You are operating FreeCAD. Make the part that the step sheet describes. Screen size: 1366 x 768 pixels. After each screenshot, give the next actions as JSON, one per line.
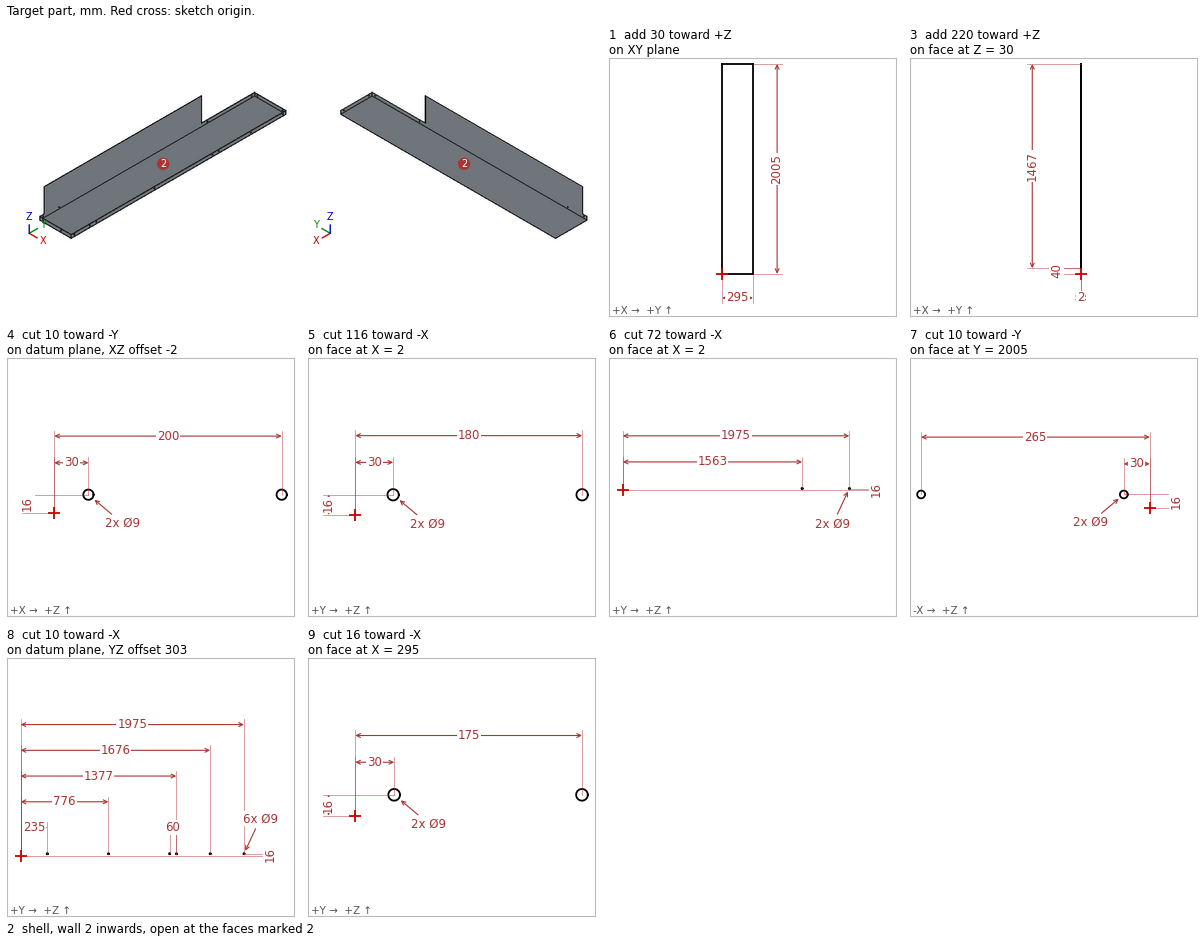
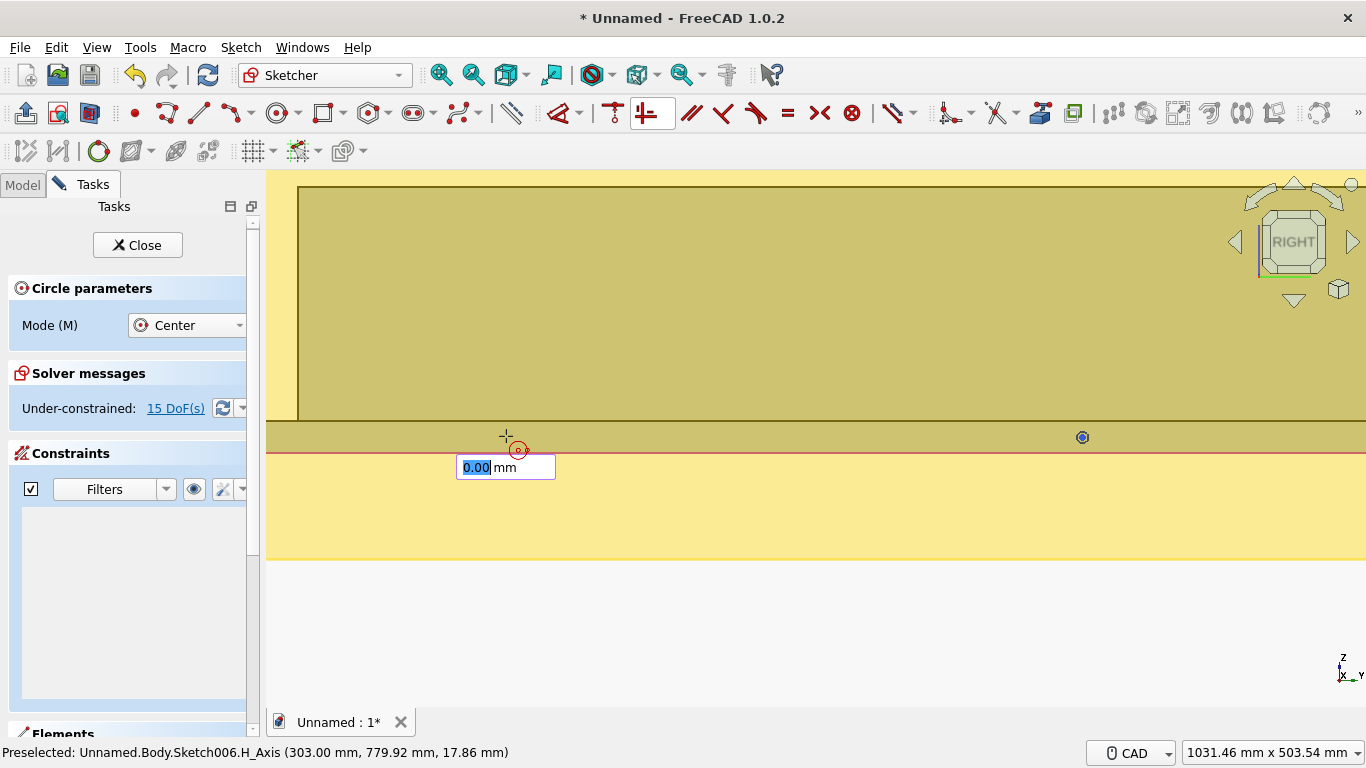
{"action": "scroll", "coordinate": [510, 433], "scroll_direction": "up", "scroll_amount": 6}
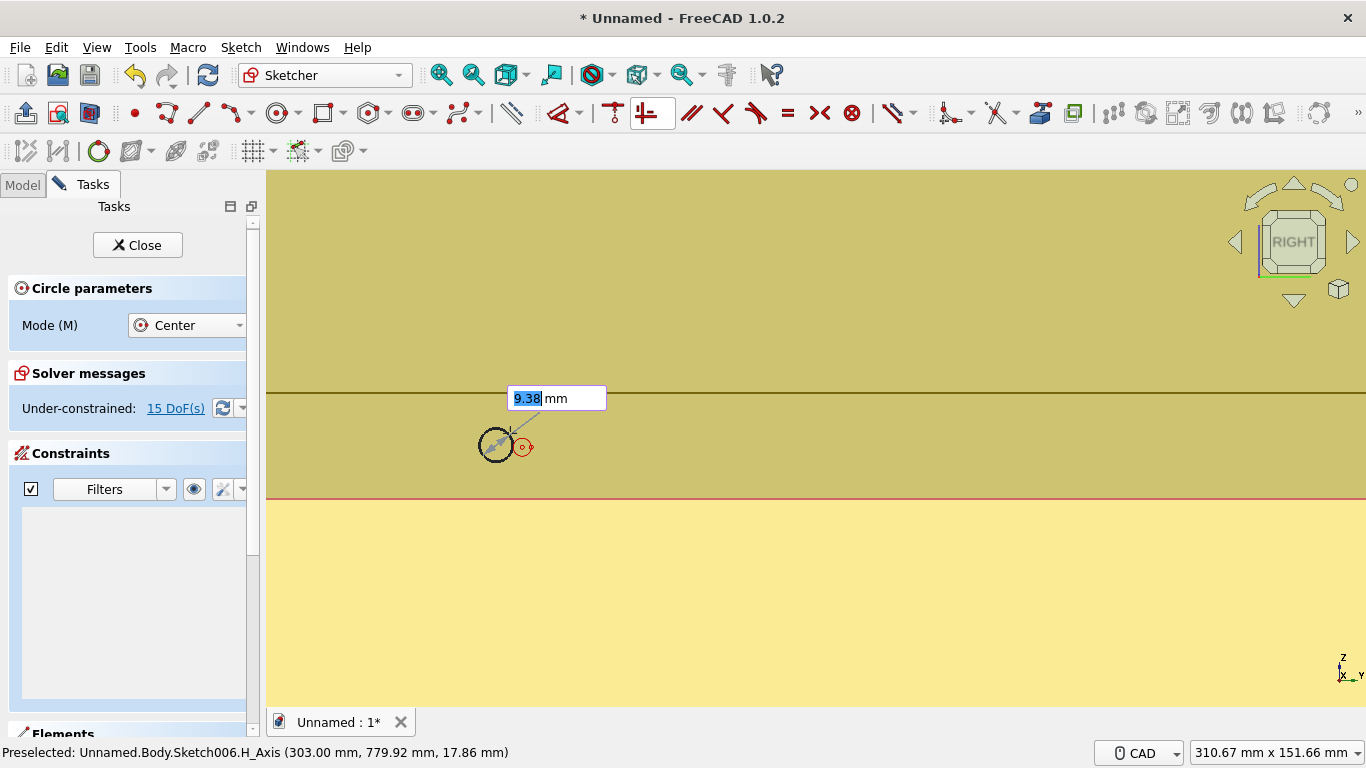
{"action": "left_click", "coordinate": [508, 431]}
{"action": "key", "text": "Escape"}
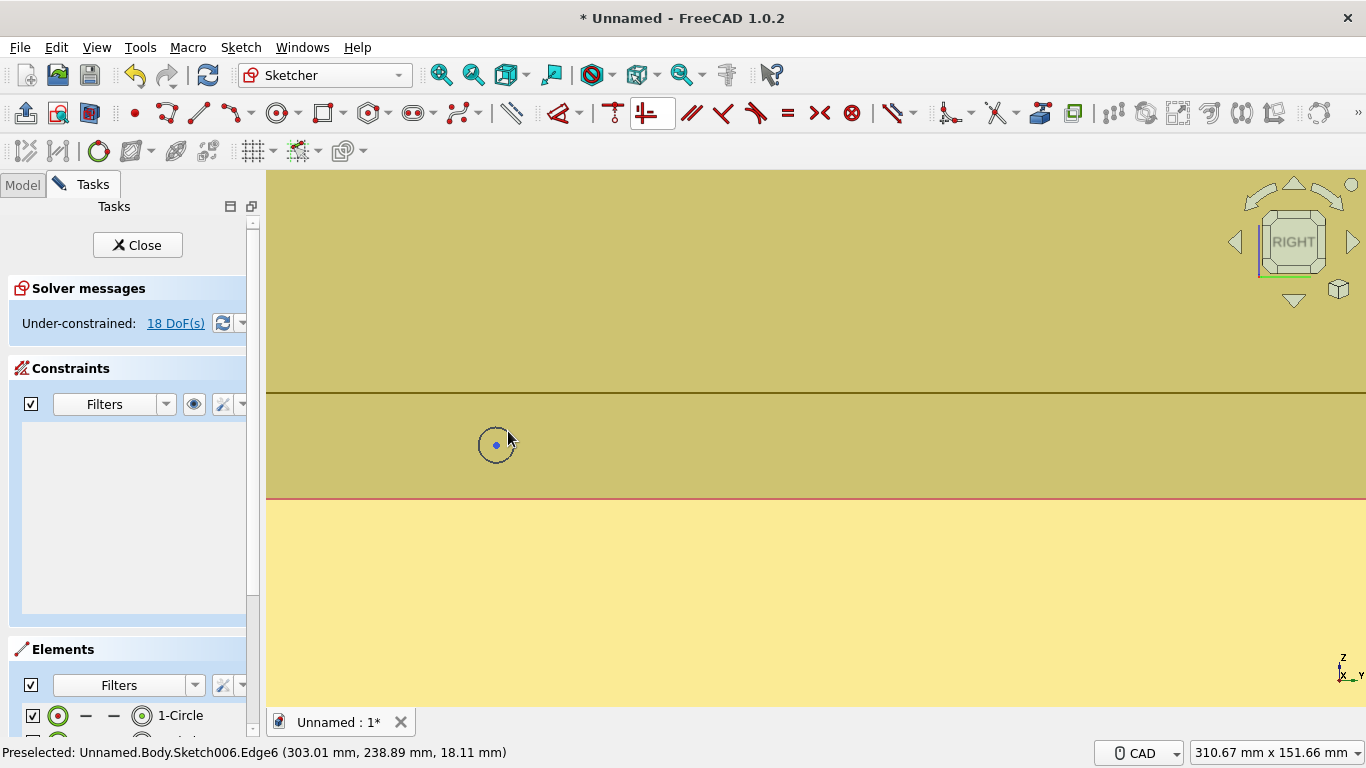
{"action": "scroll", "coordinate": [506, 436], "scroll_direction": "down", "scroll_amount": 12}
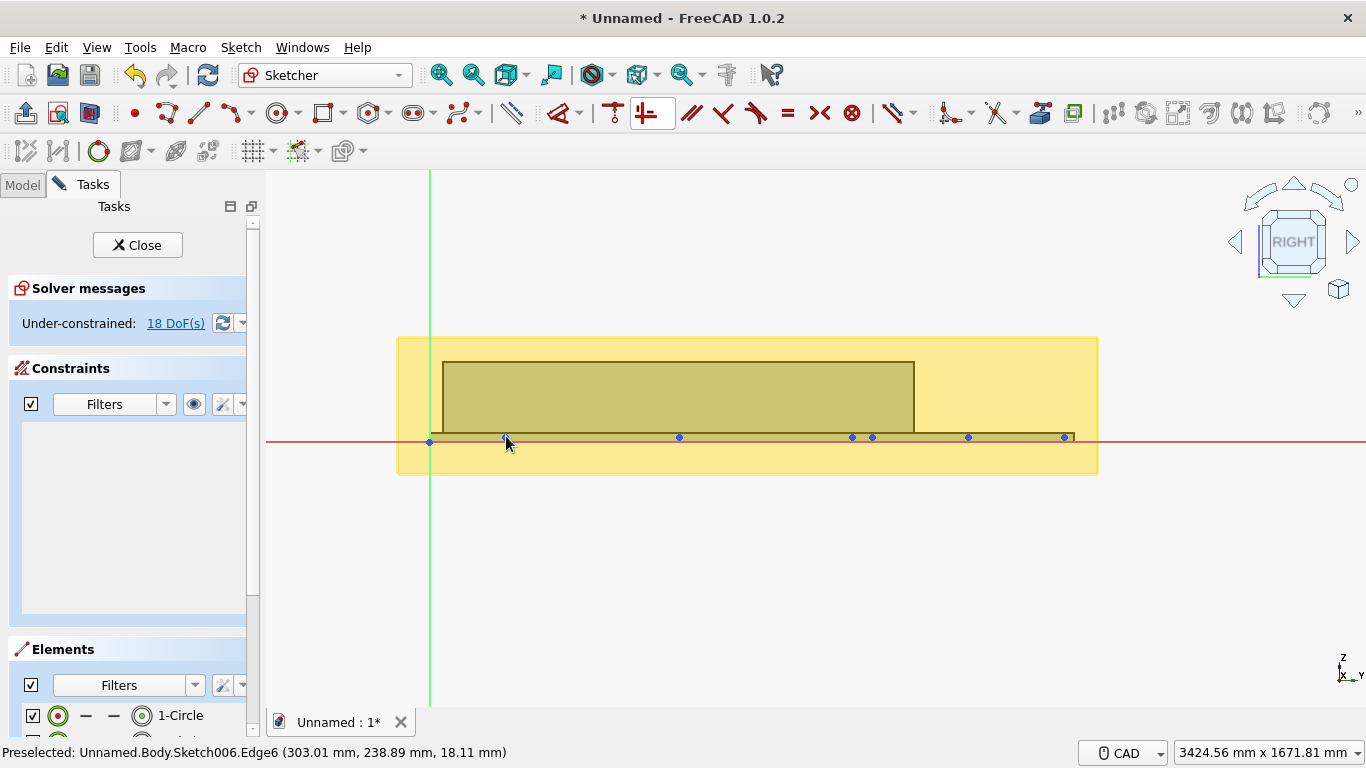
{"action": "scroll", "coordinate": [1065, 436], "scroll_direction": "up", "scroll_amount": 11}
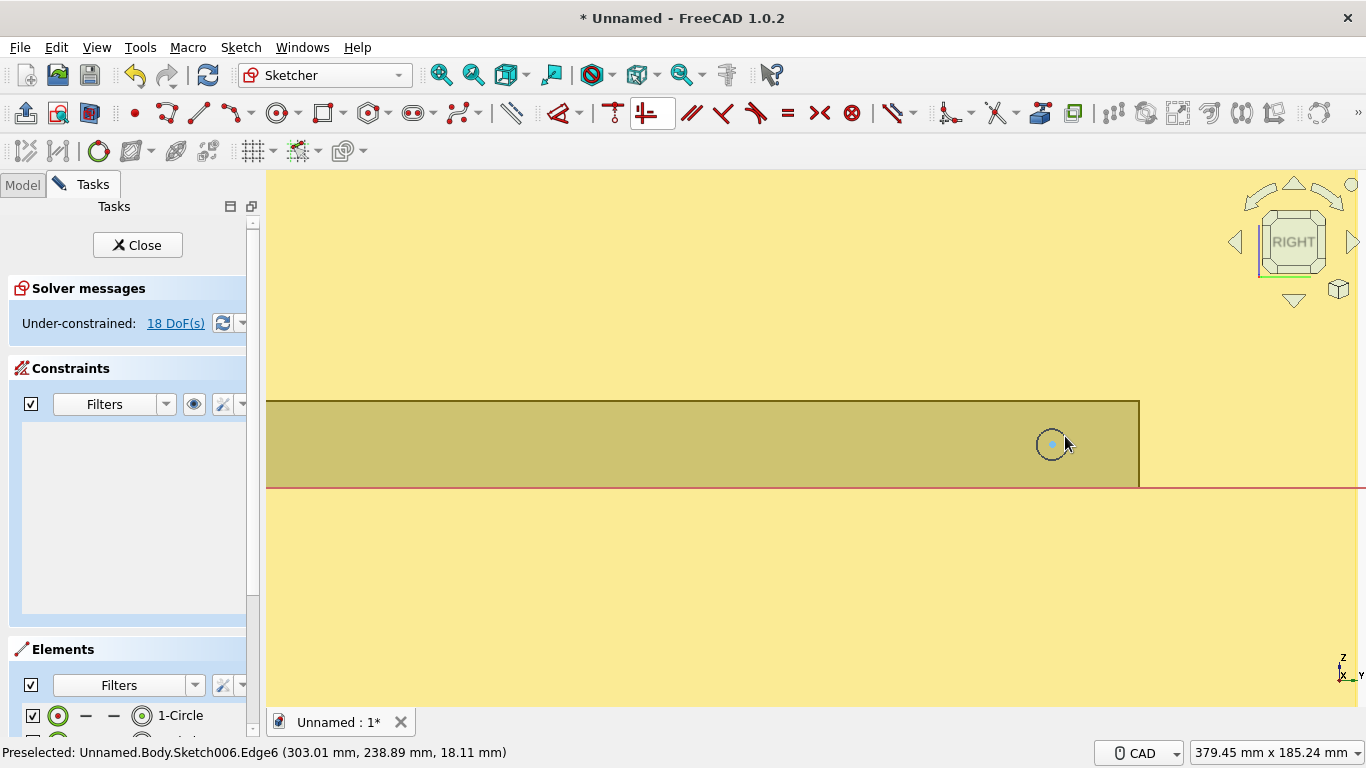
{"action": "left_click", "coordinate": [1063, 434]}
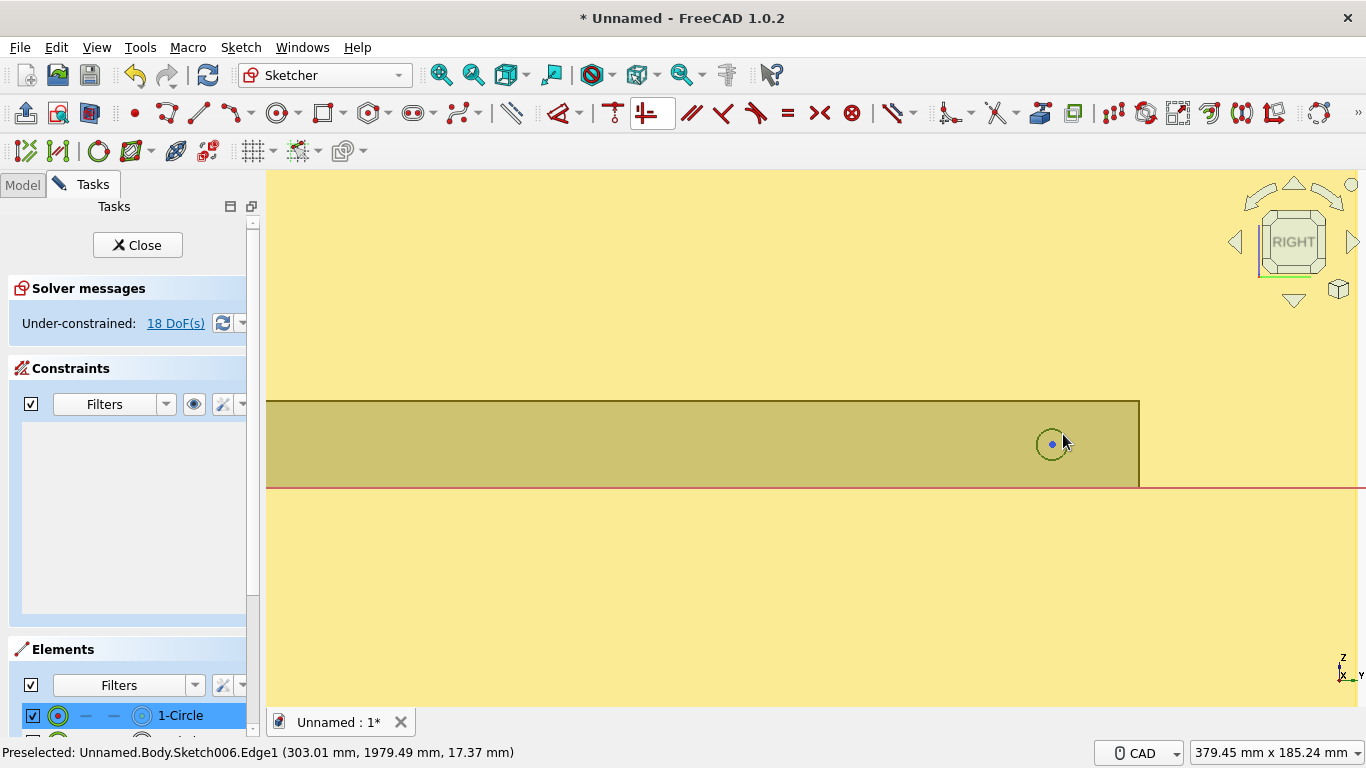
{"action": "scroll", "coordinate": [1065, 436], "scroll_direction": "down", "scroll_amount": 11}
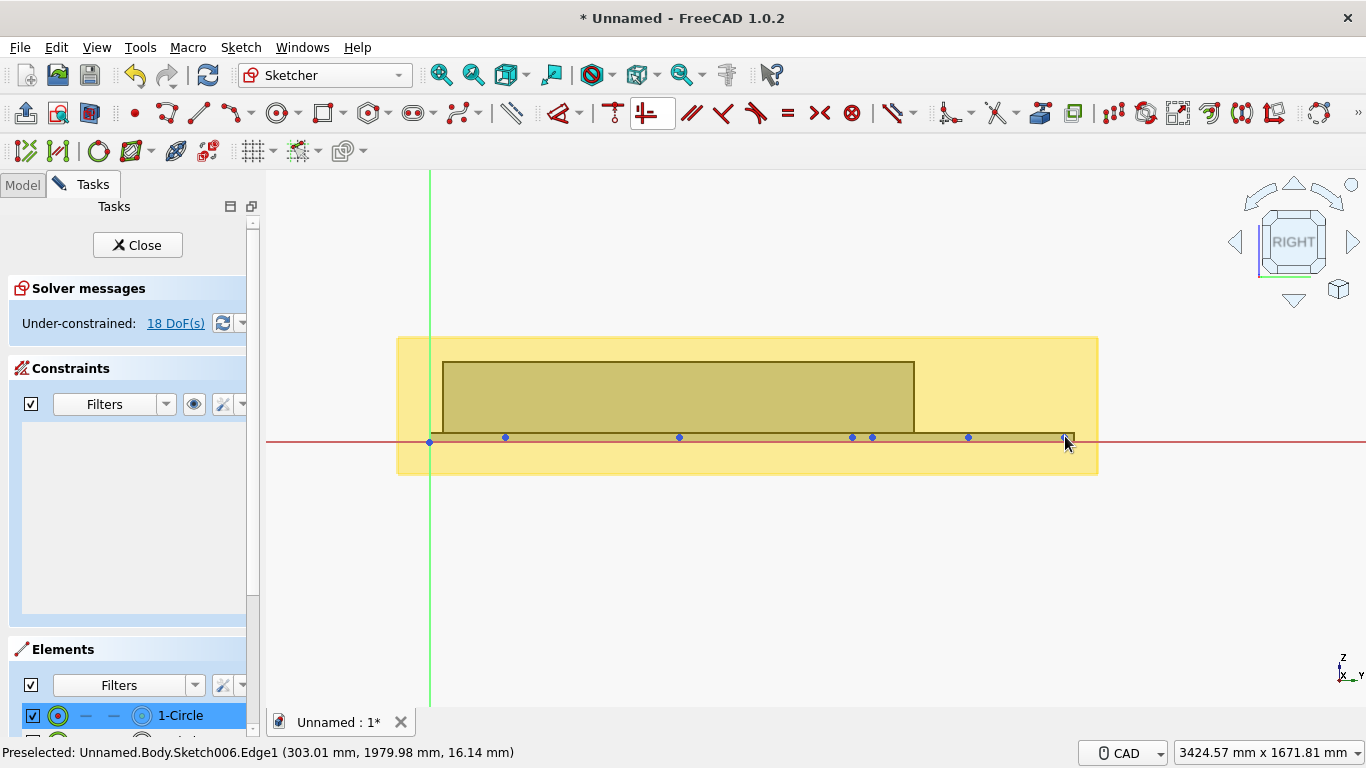
{"action": "scroll", "coordinate": [969, 436], "scroll_direction": "up", "scroll_amount": 11}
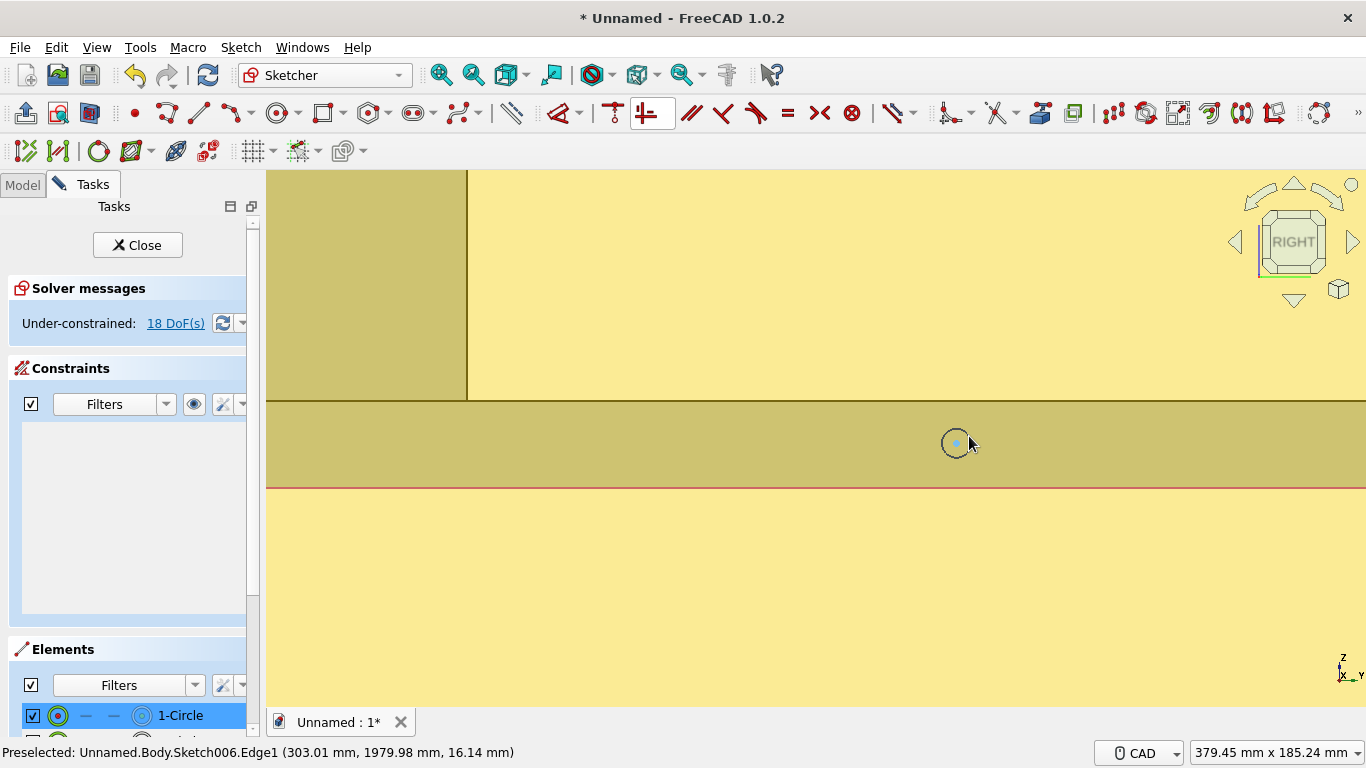
{"action": "left_click", "coordinate": [967, 433]}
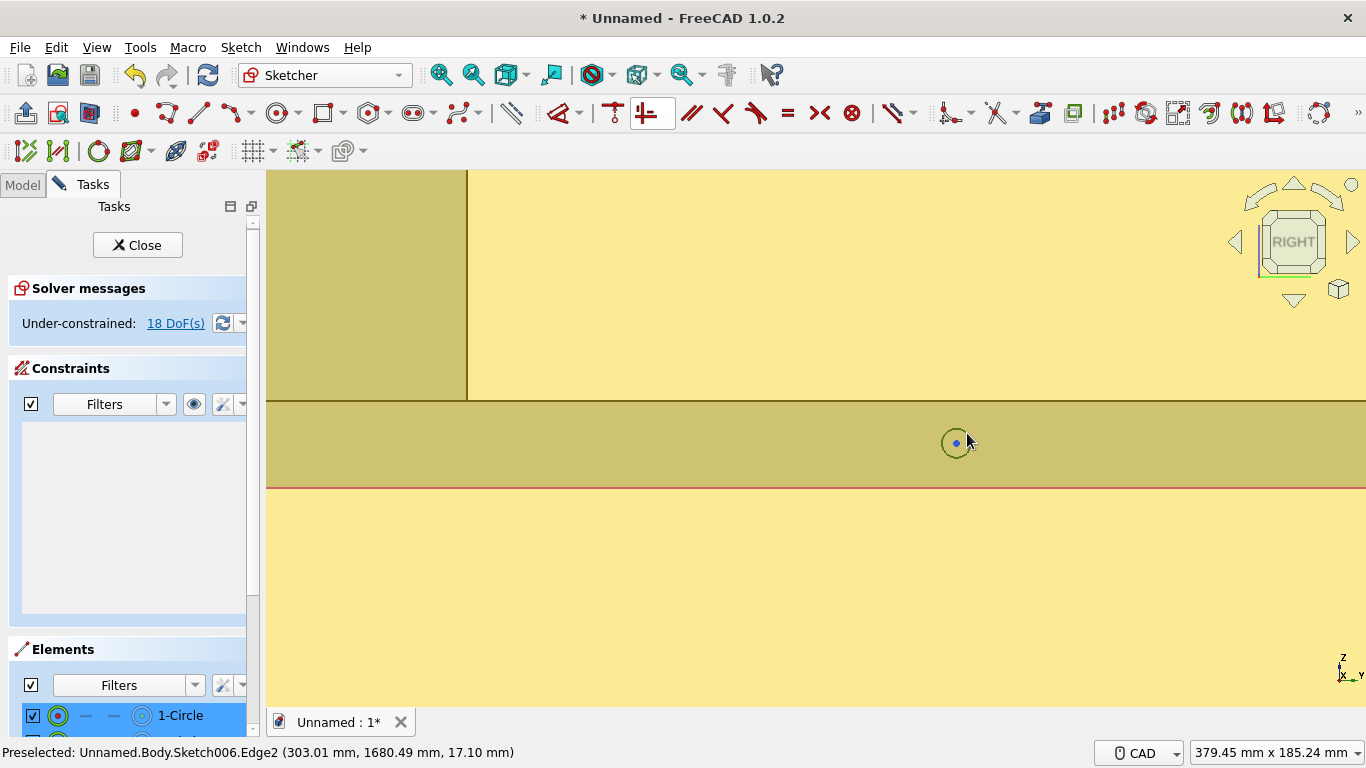
{"action": "scroll", "coordinate": [969, 436], "scroll_direction": "down", "scroll_amount": 11}